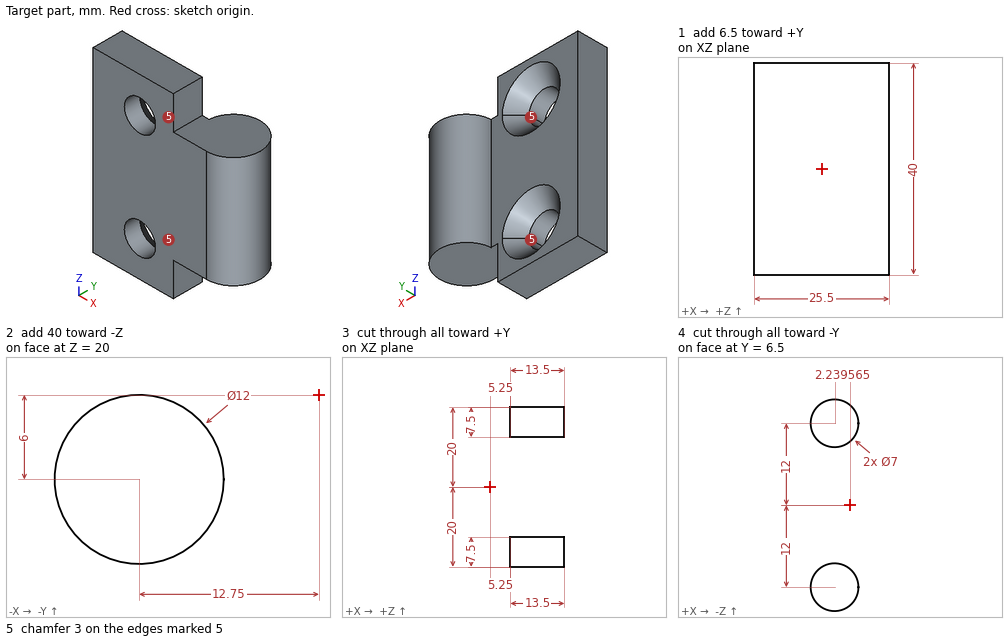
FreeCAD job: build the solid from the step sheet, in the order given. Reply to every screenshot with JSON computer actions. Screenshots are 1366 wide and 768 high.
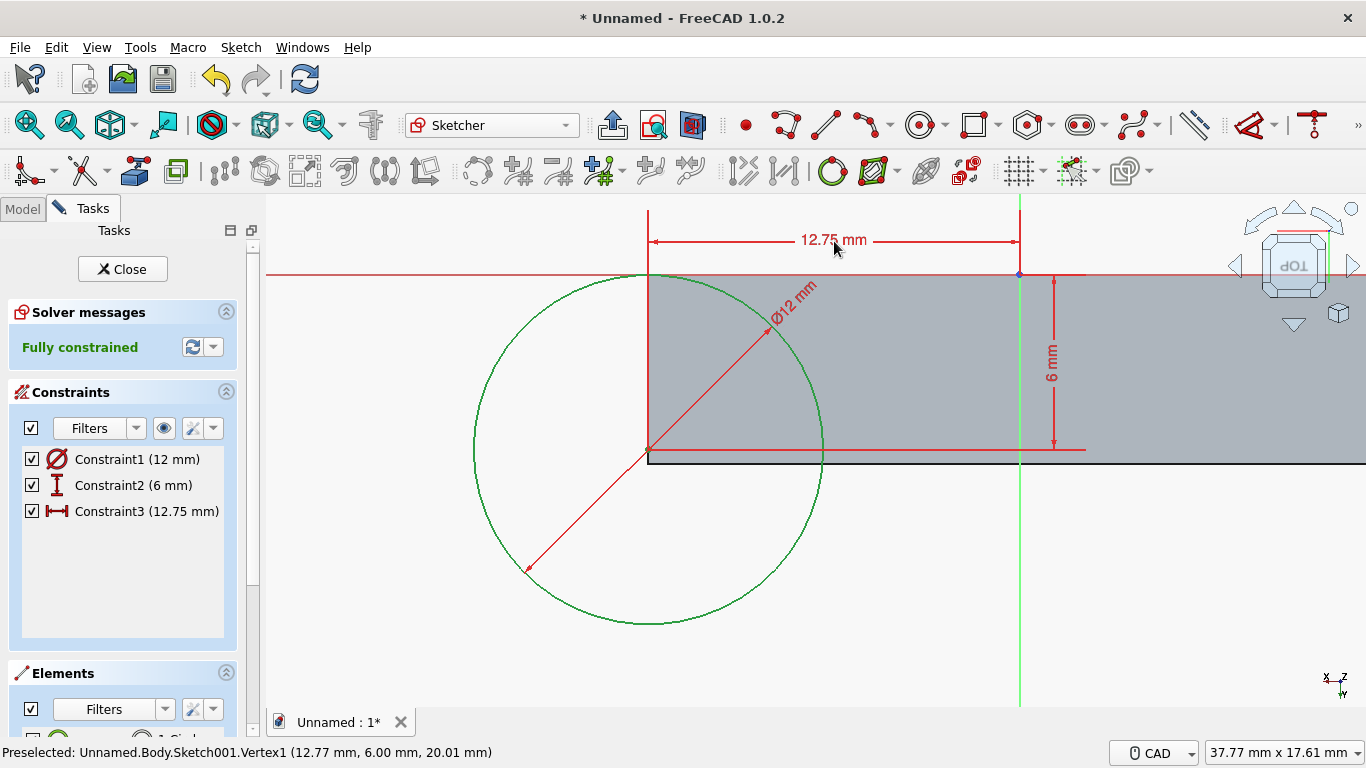
{"action": "left_click", "coordinate": [123, 269]}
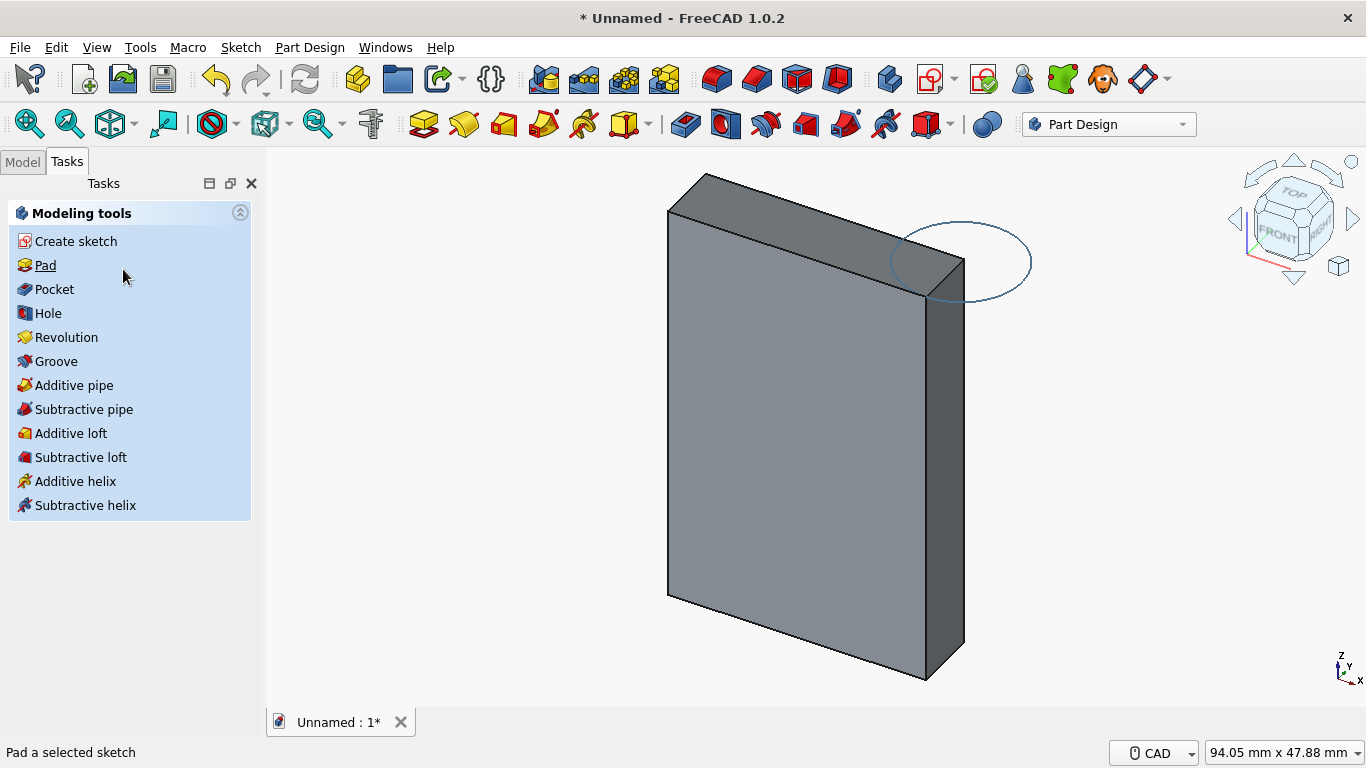
{"action": "left_click", "coordinate": [424, 124]}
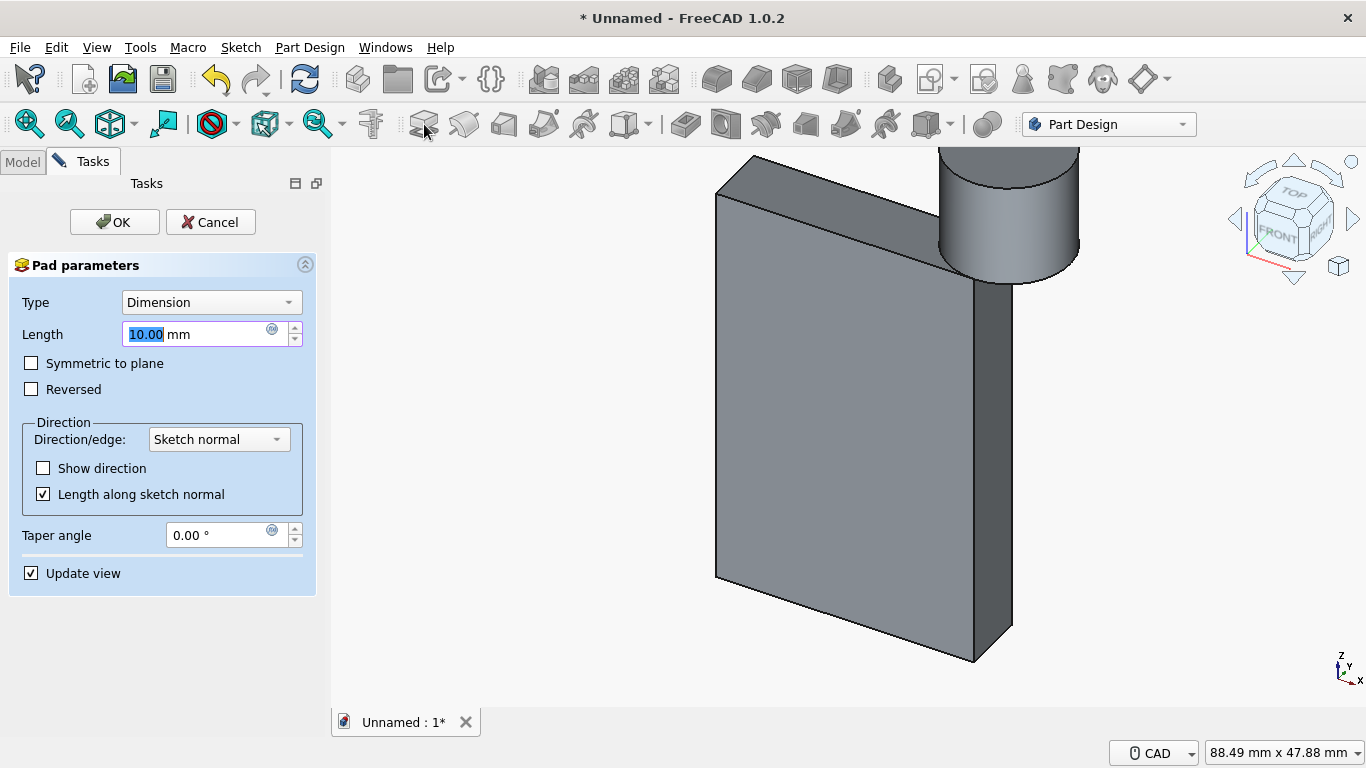
{"action": "type", "text": "40"}
{"action": "key", "text": "Tab"}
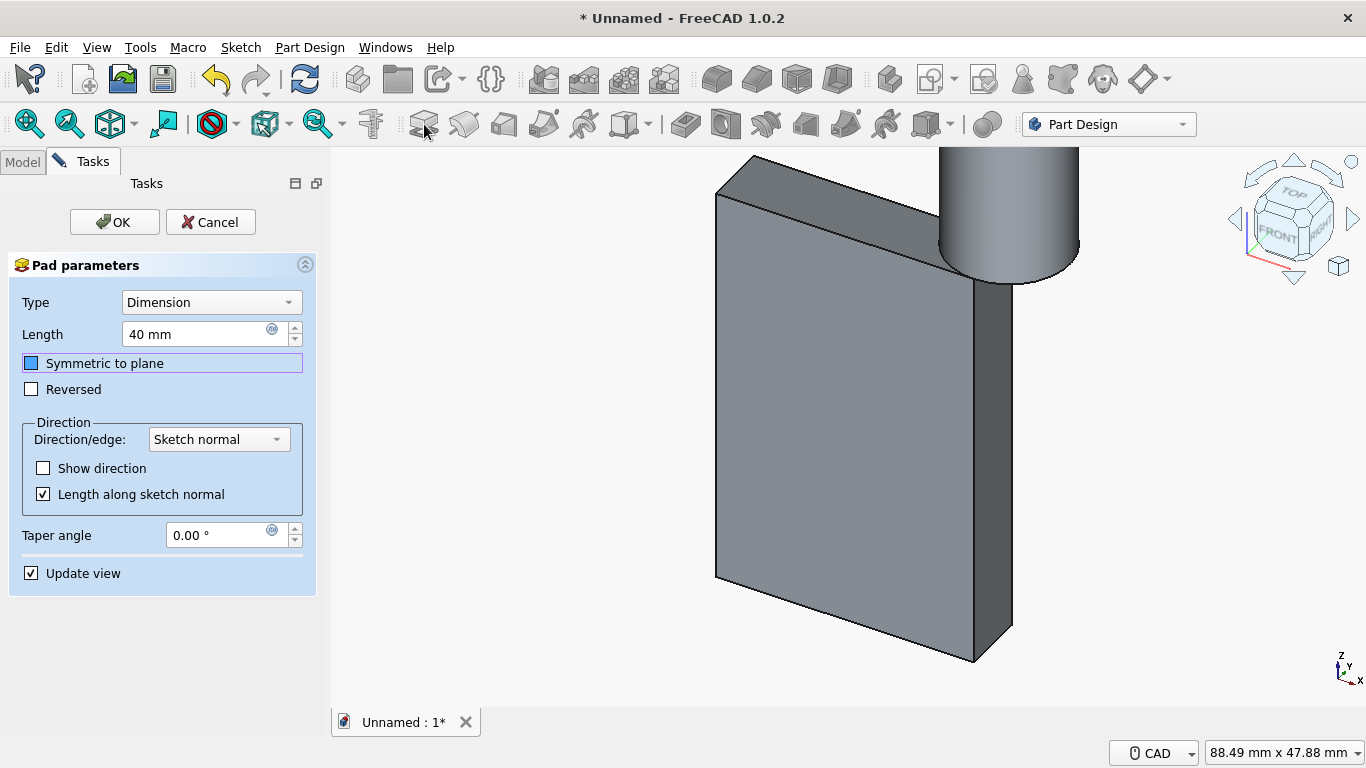
{"action": "left_click", "coordinate": [30, 389]}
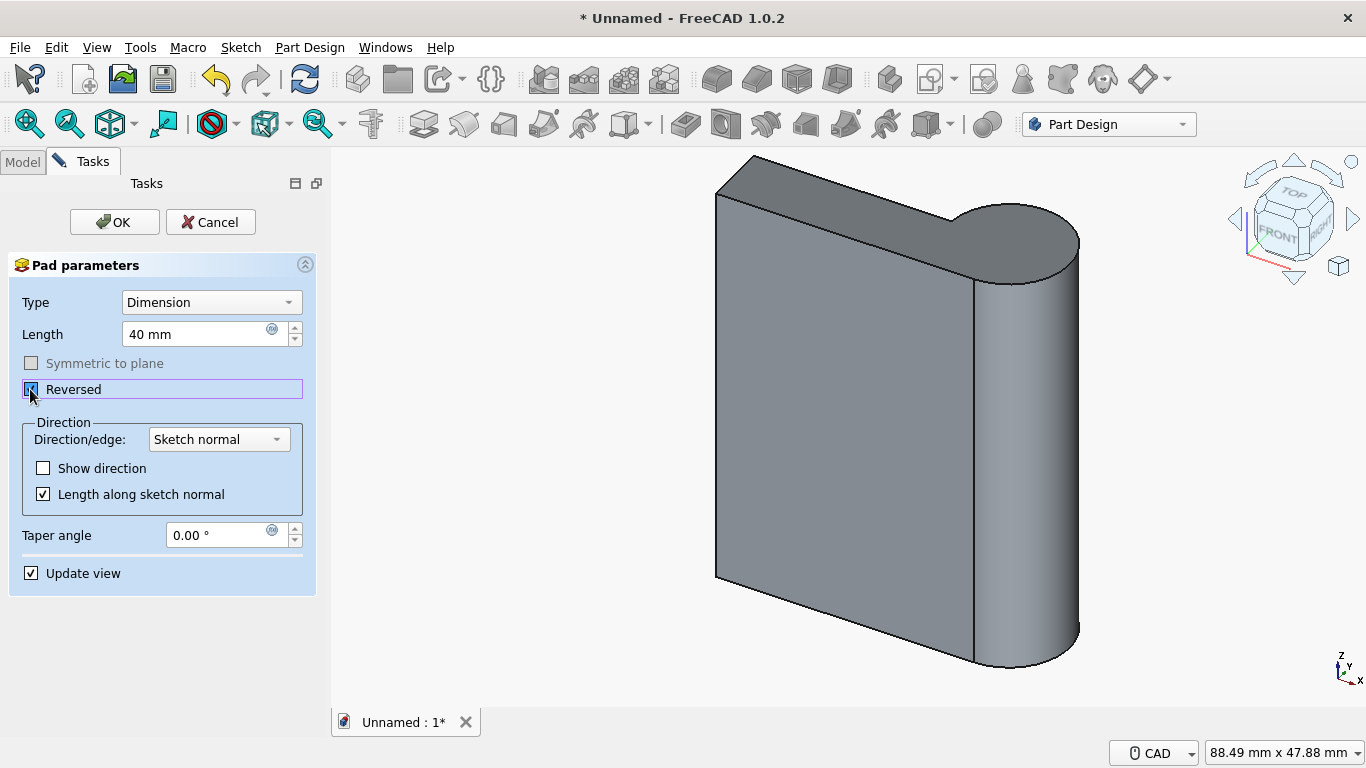
{"action": "left_click", "coordinate": [115, 222]}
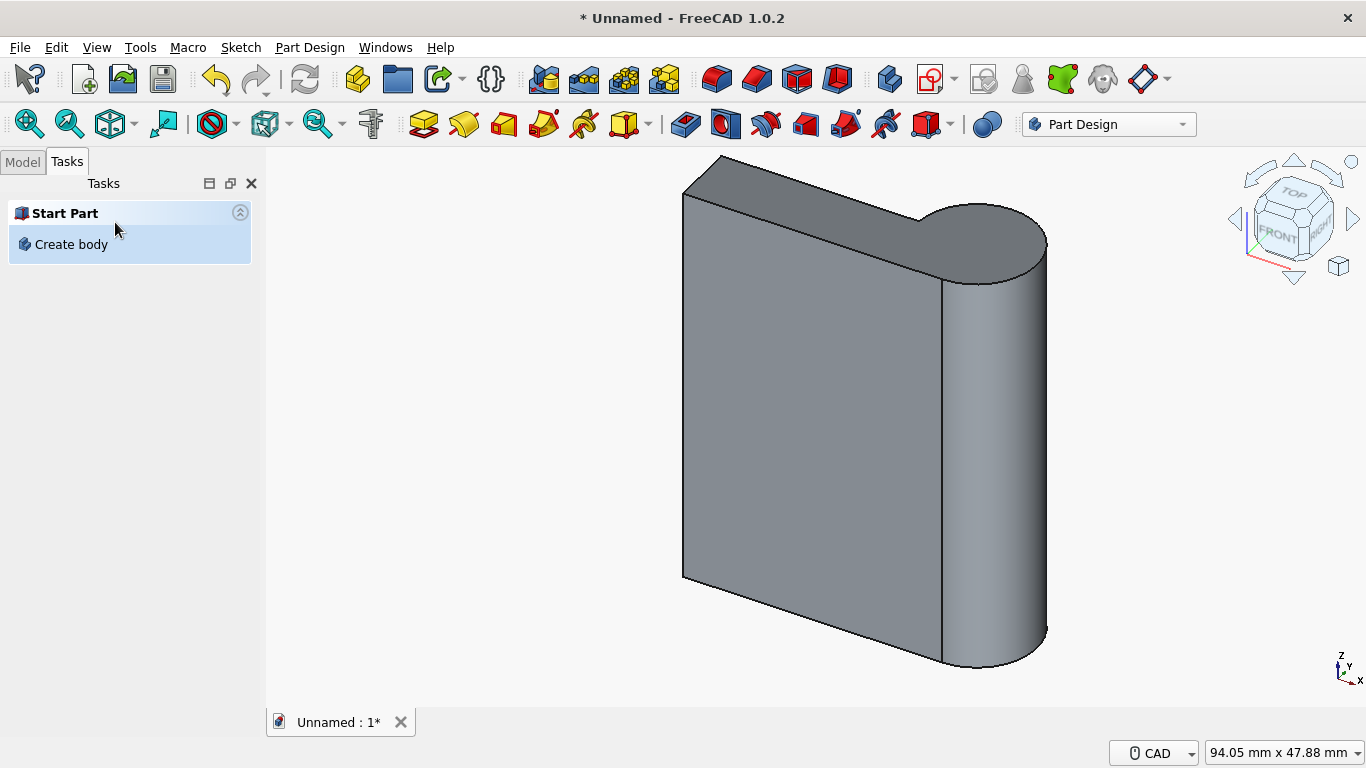
{"action": "left_click", "coordinate": [30, 124]}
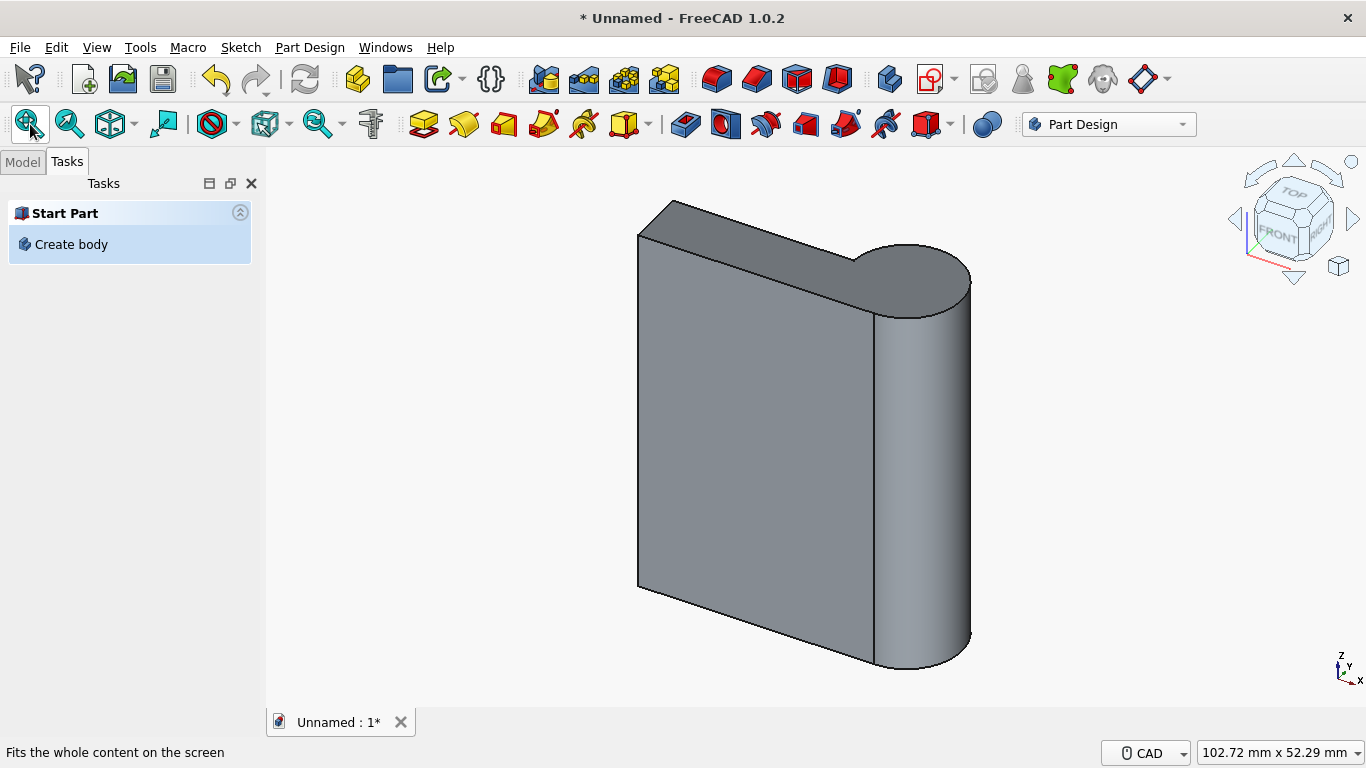
{"action": "left_click", "coordinate": [930, 80]}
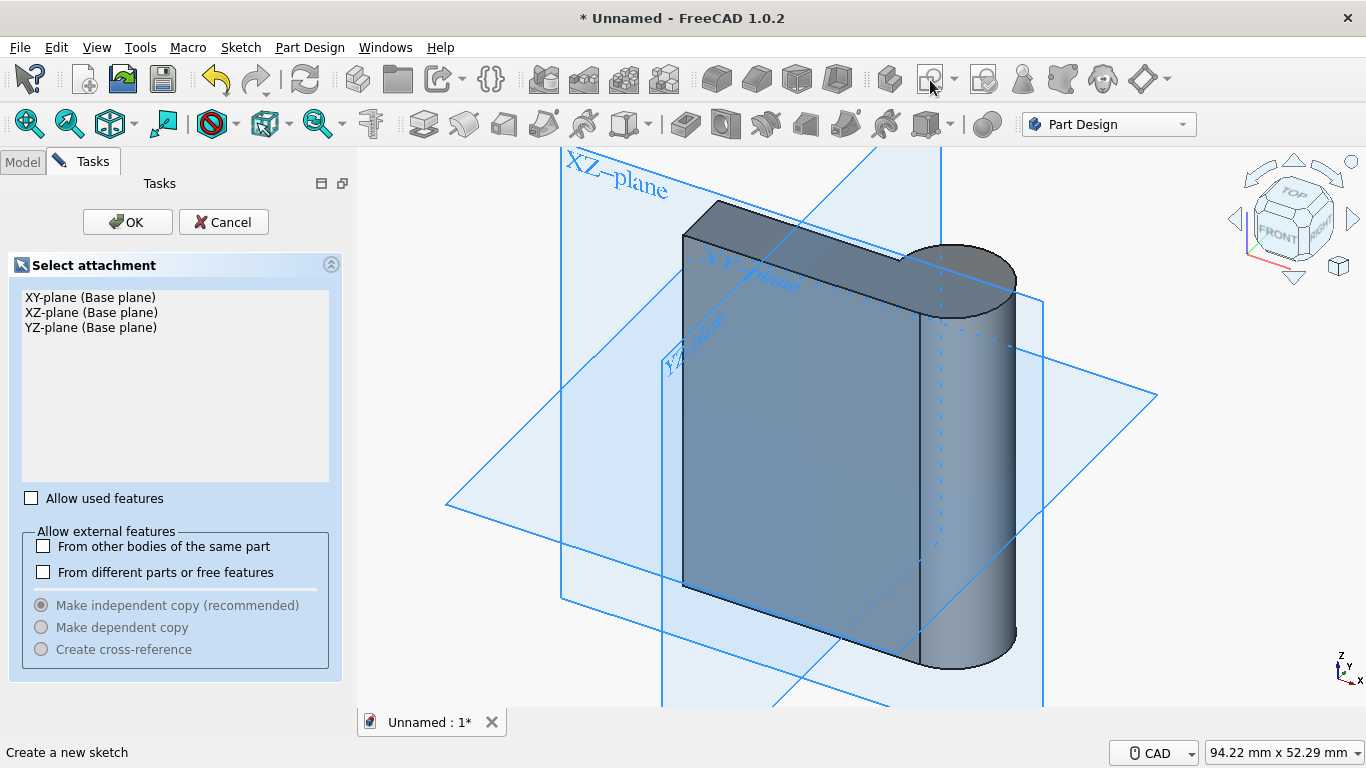
{"action": "left_click", "coordinate": [82, 312]}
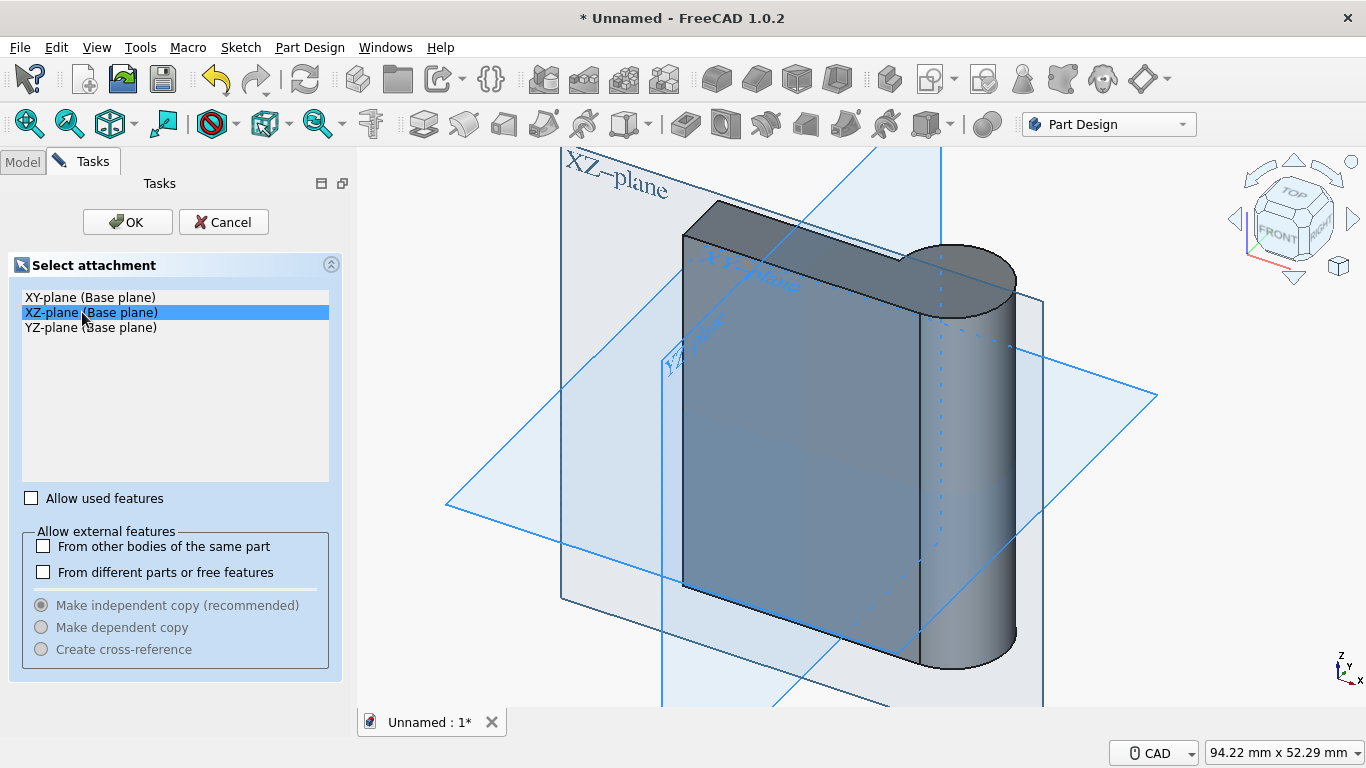
{"action": "left_click", "coordinate": [128, 222]}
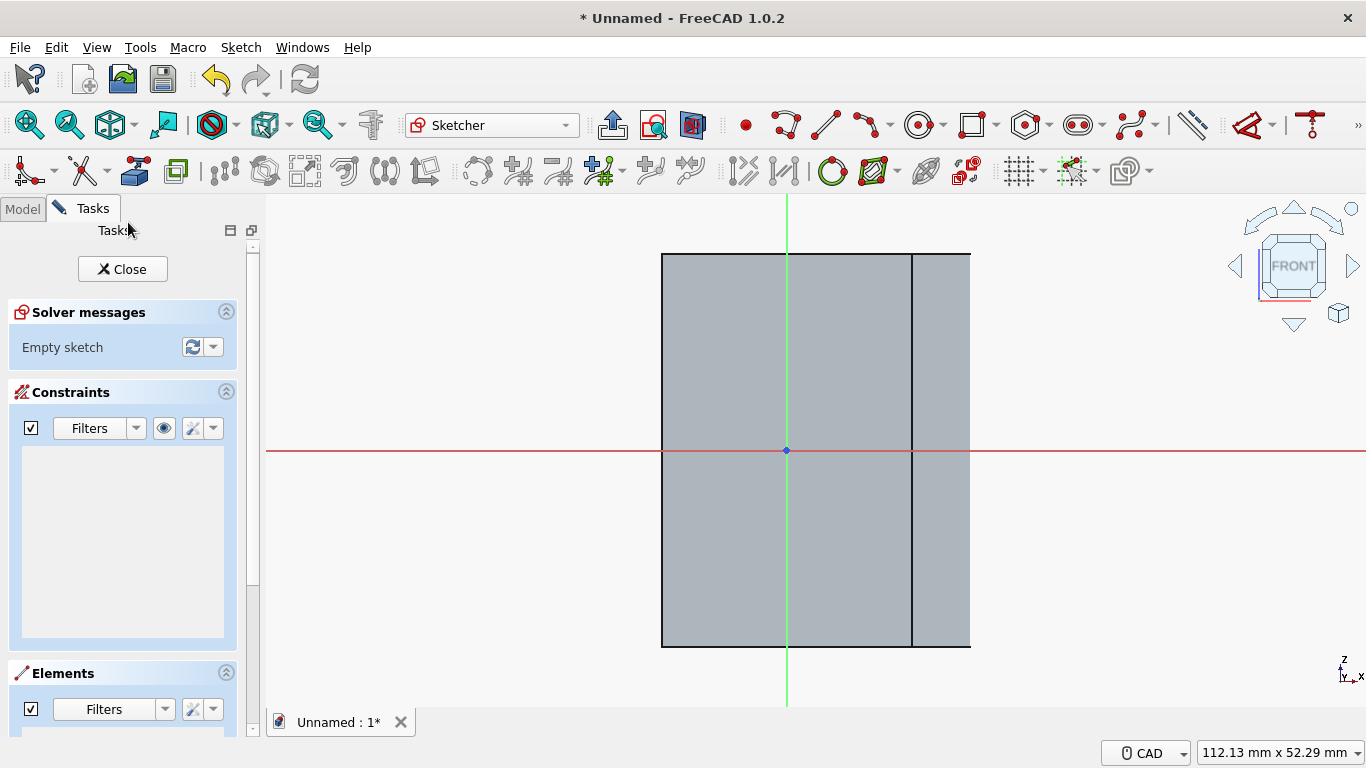
{"action": "left_click", "coordinate": [972, 126]}